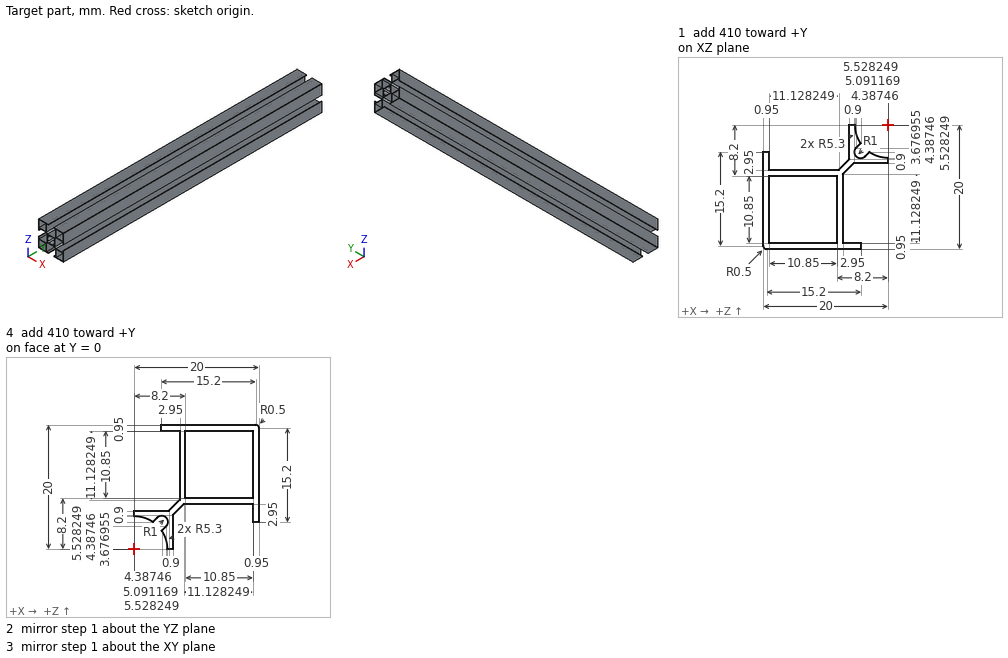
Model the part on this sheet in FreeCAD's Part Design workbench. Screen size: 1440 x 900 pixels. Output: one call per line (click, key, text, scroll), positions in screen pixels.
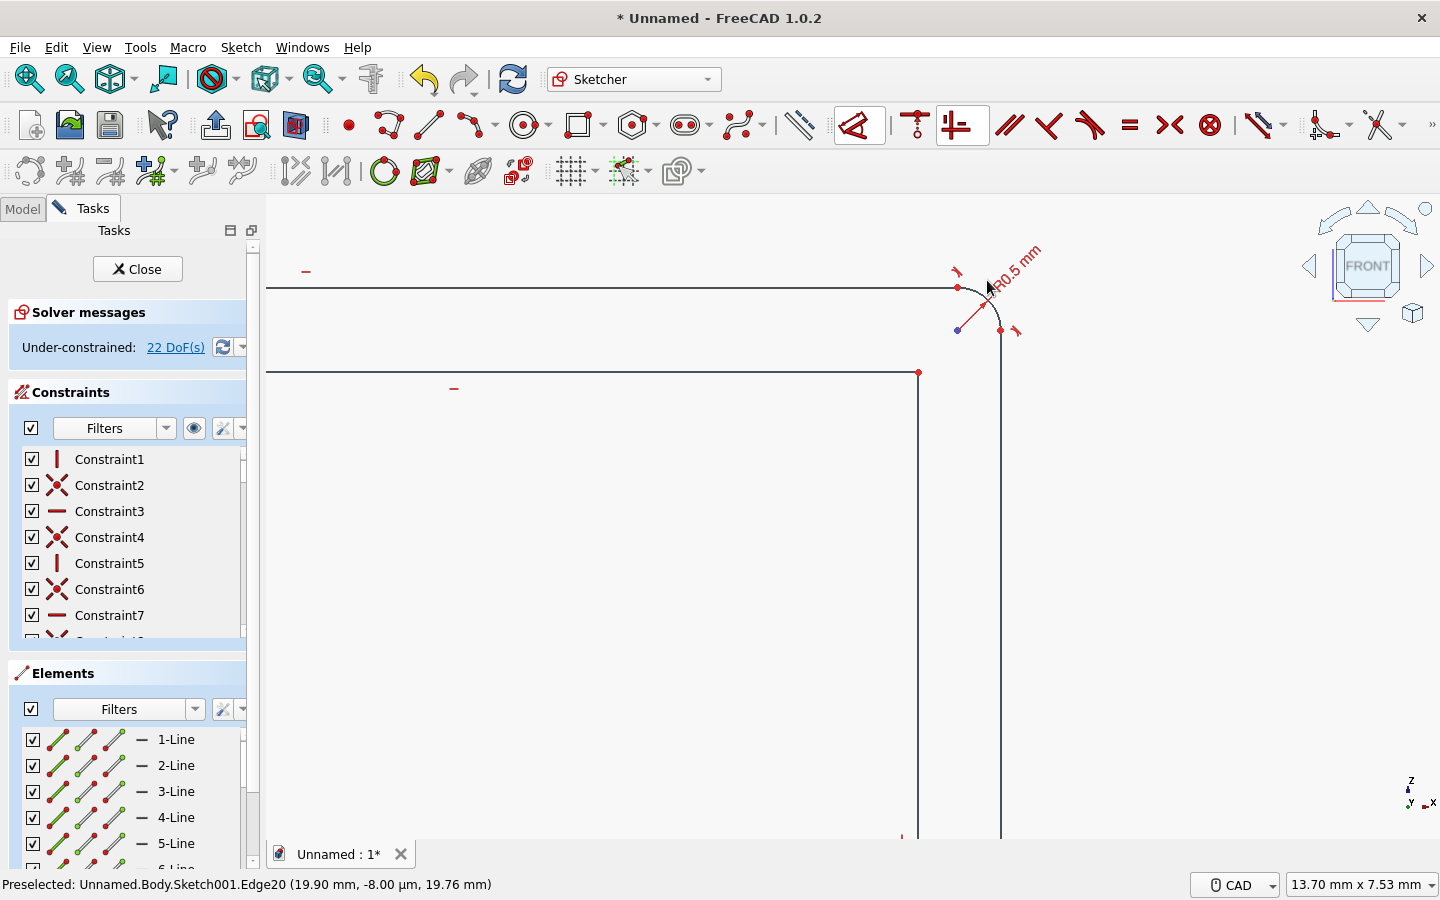
scroll(994, 311, down, 7)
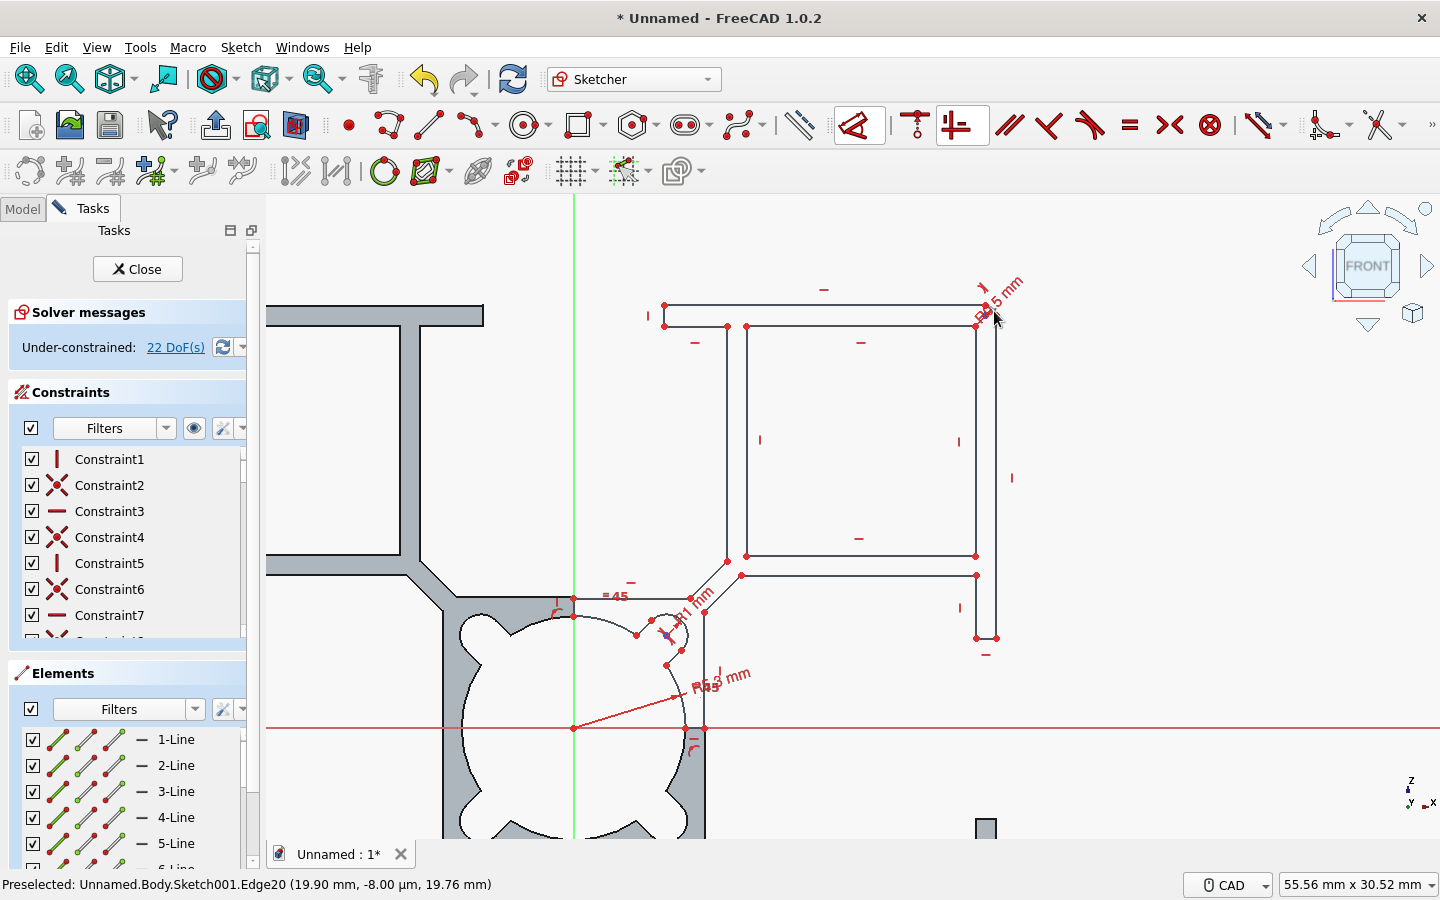
scroll(699, 728, up, 5)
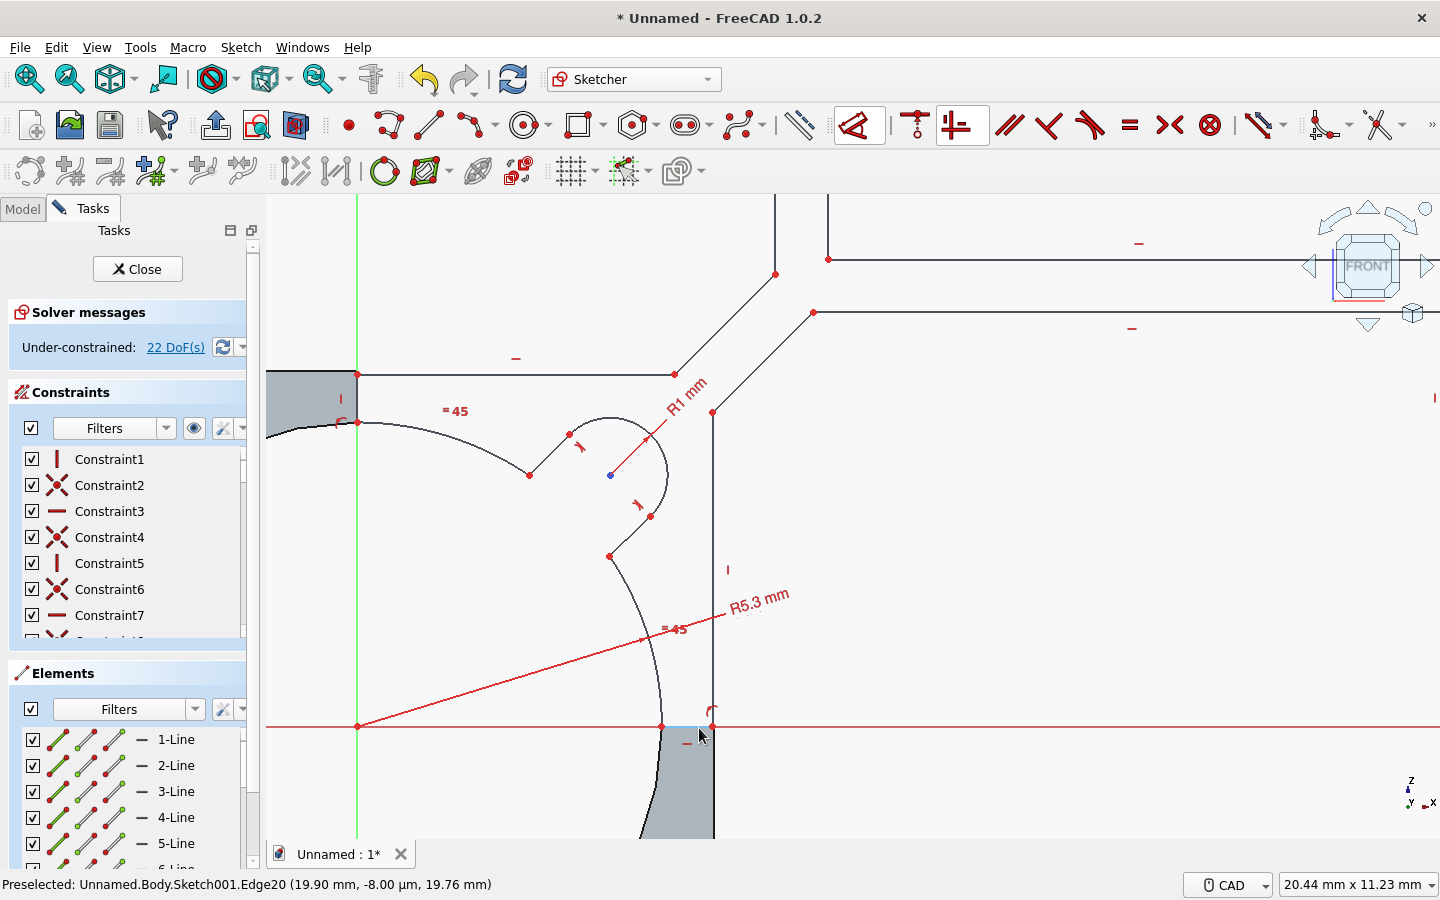
click(697, 727)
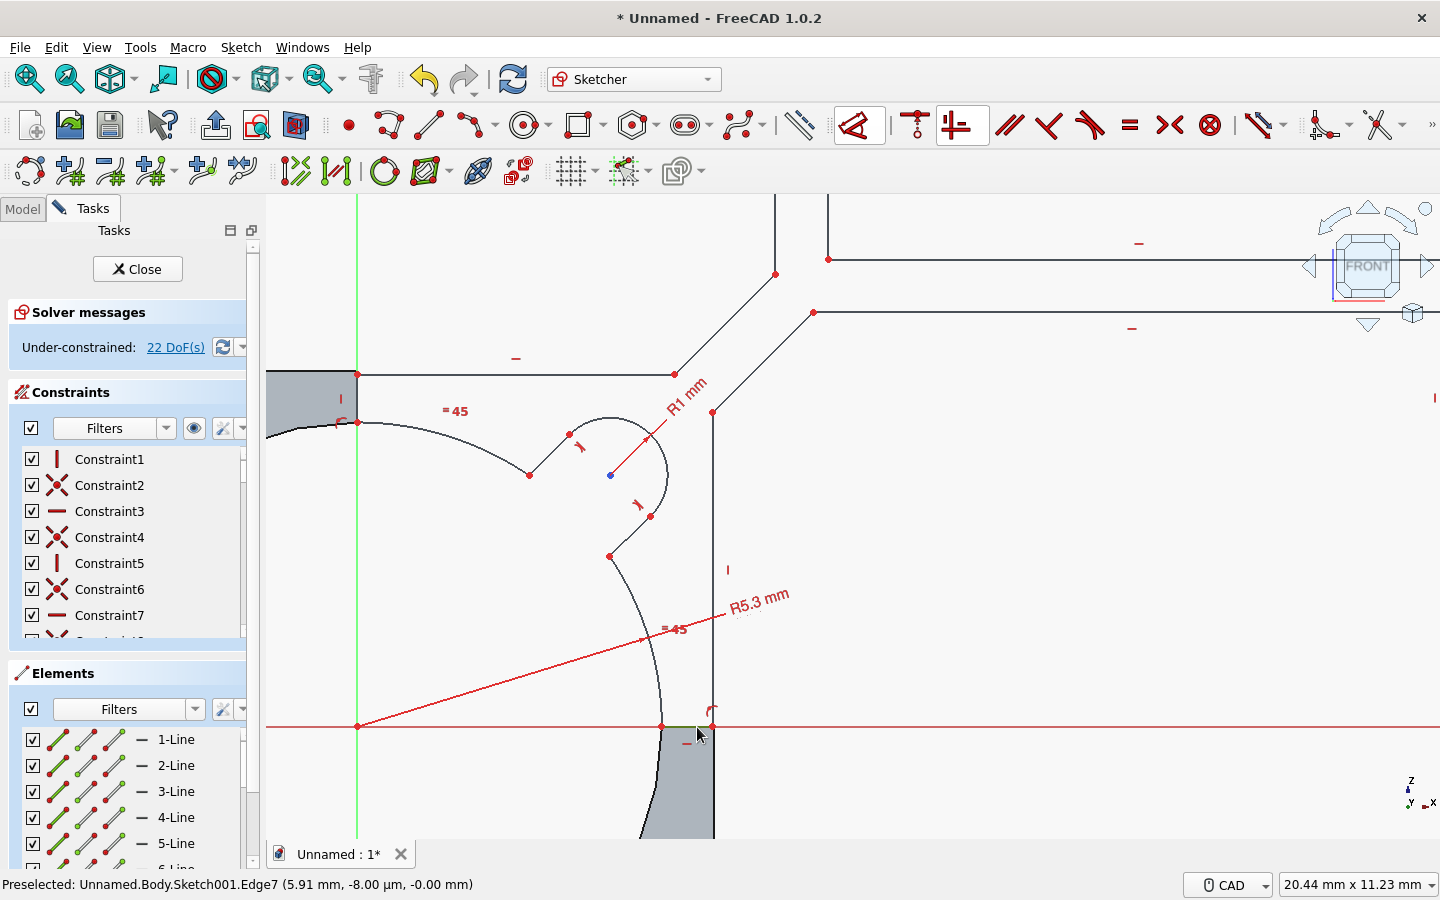
click(880, 126)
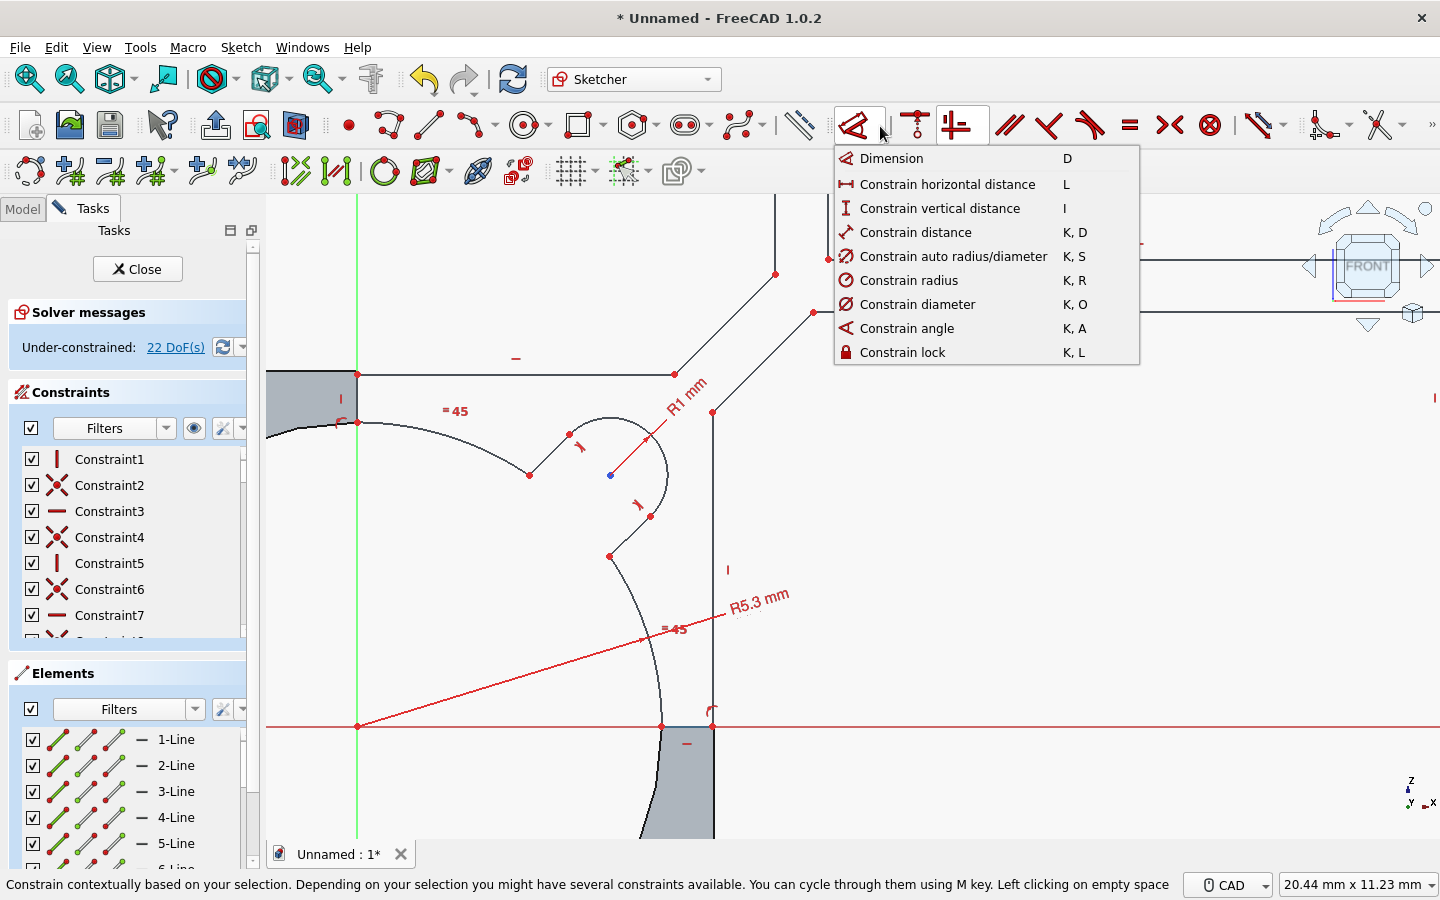
click(987, 184)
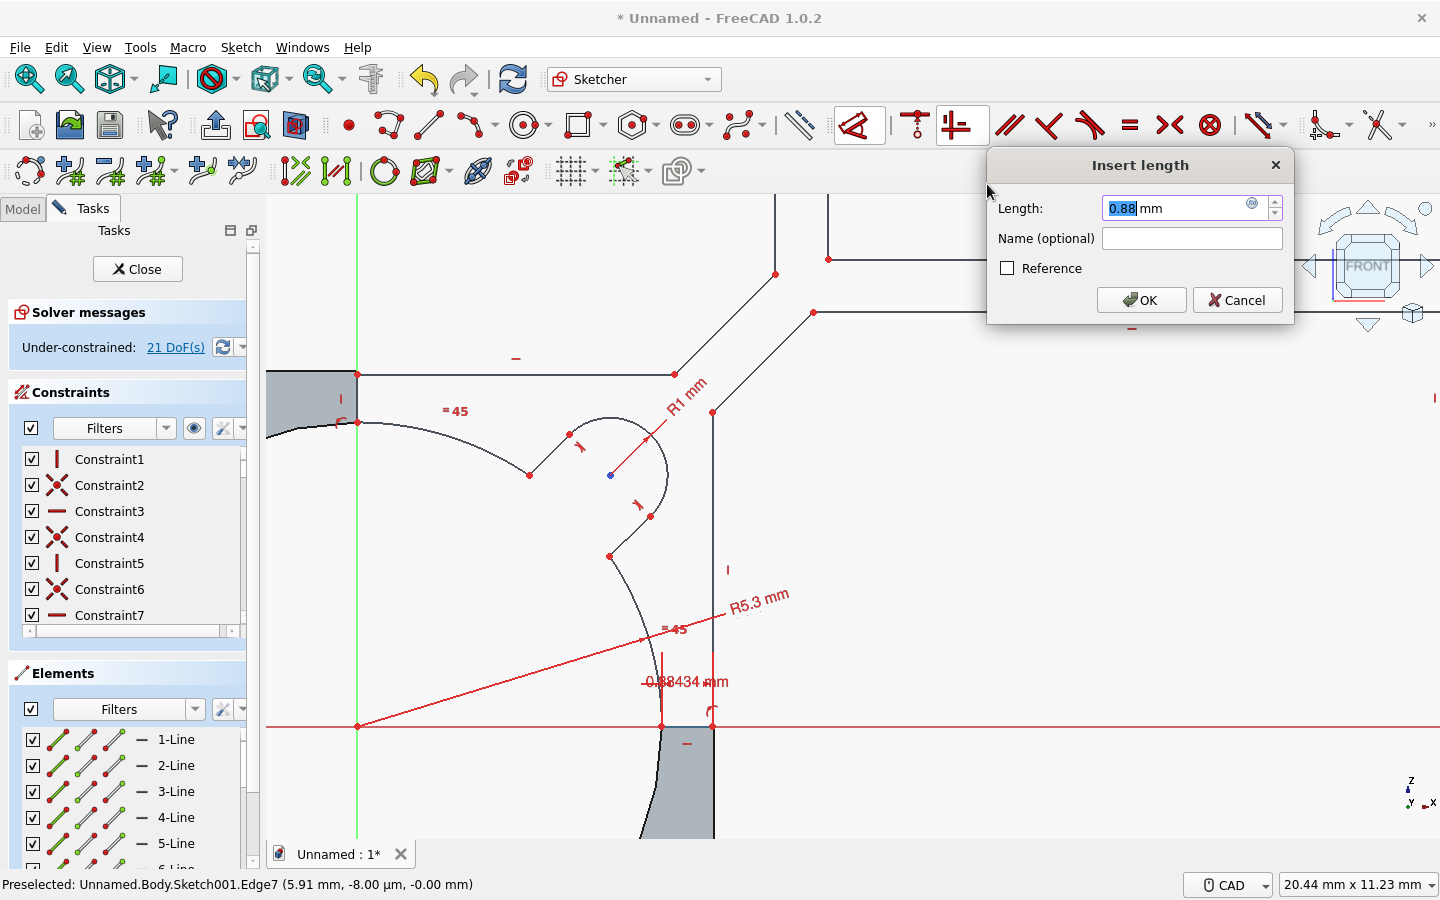
text(0.9)
key(Return)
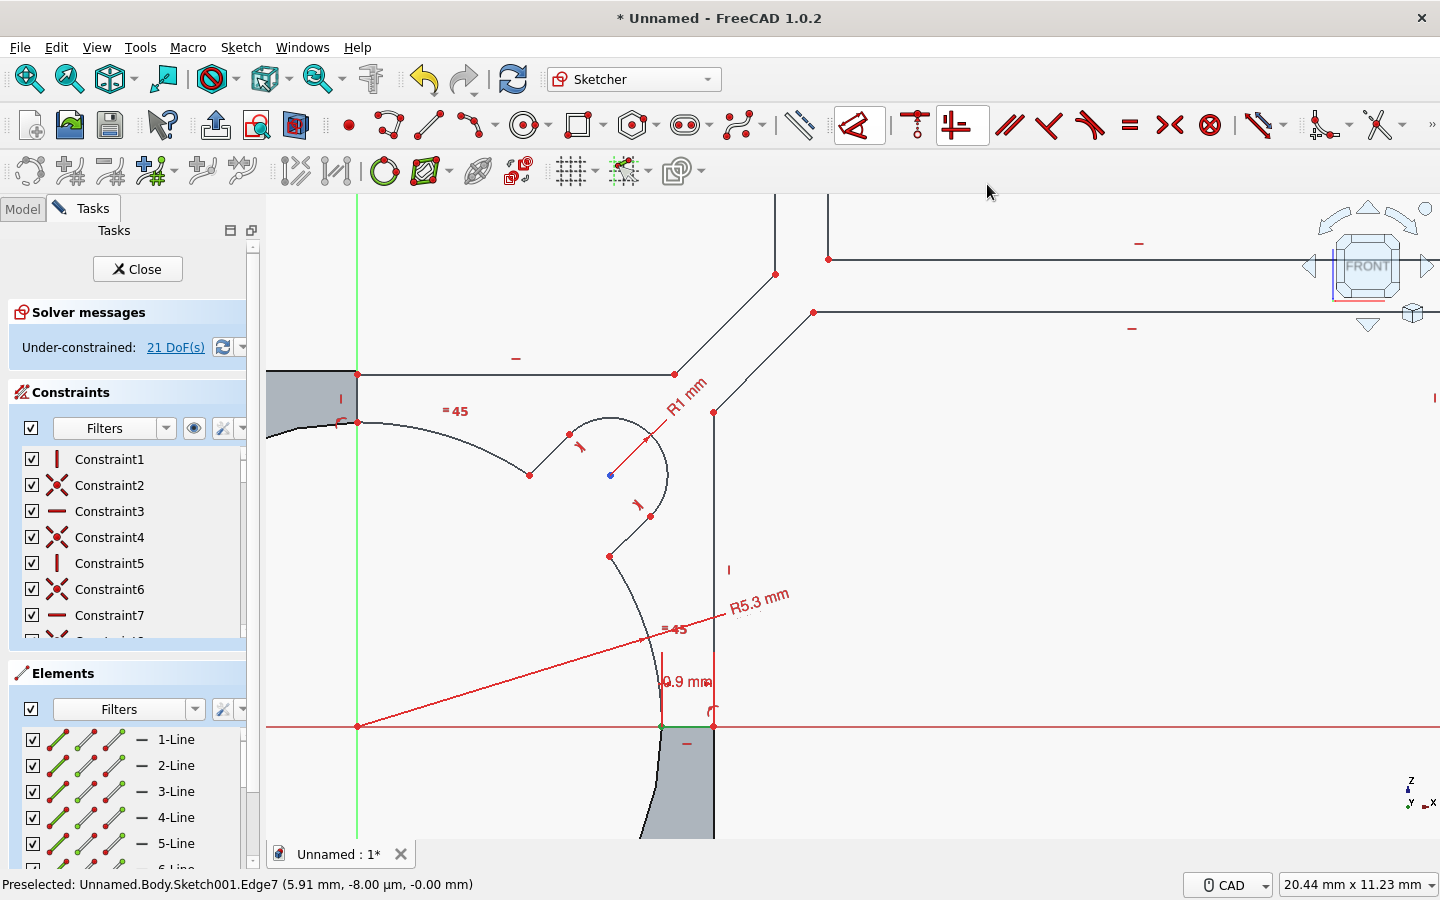
click(357, 408)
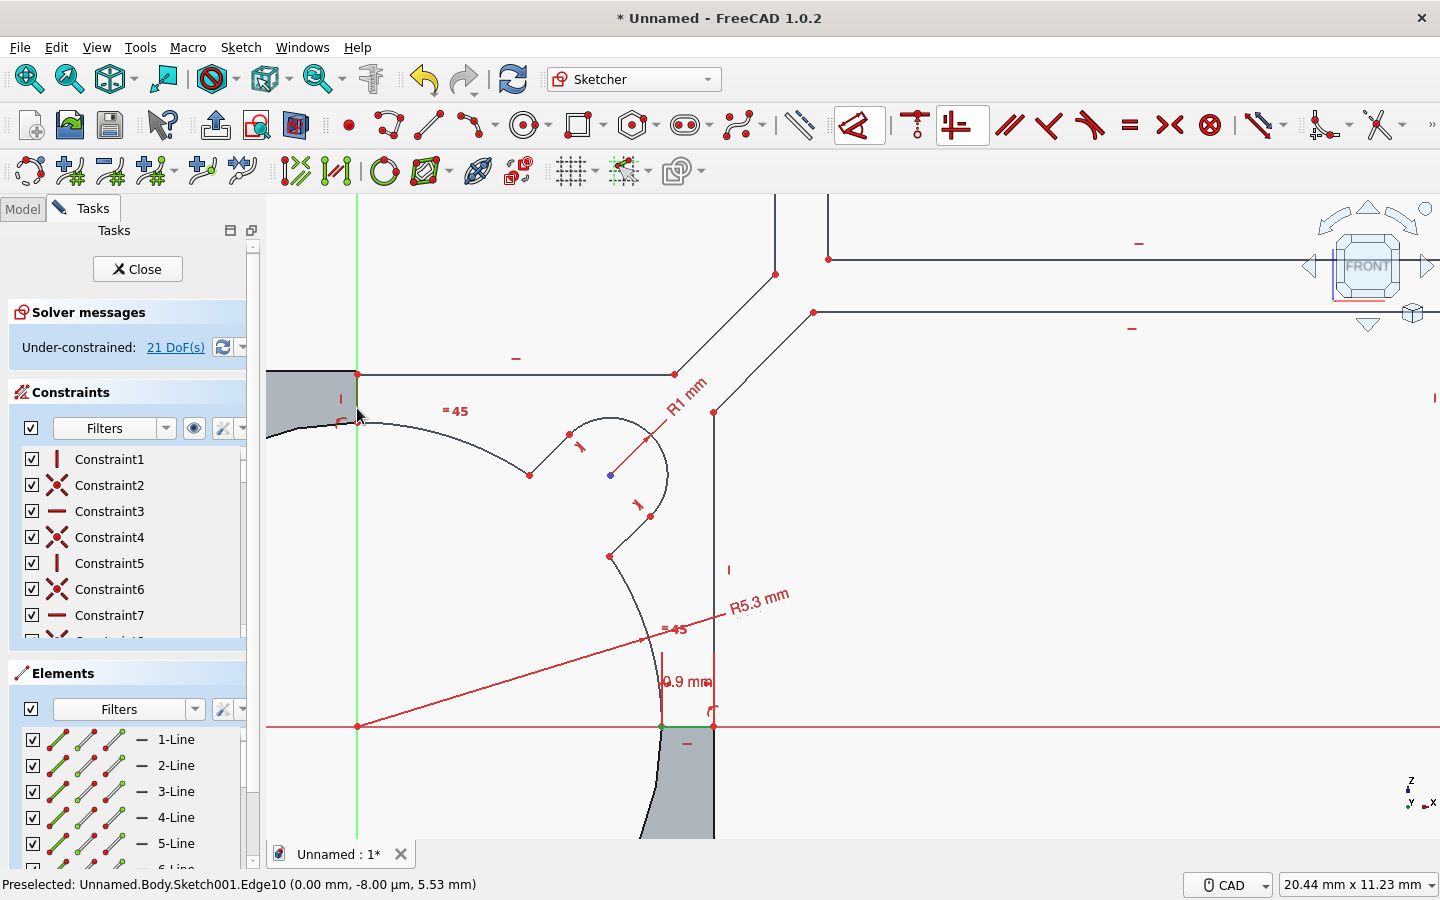
key(i)